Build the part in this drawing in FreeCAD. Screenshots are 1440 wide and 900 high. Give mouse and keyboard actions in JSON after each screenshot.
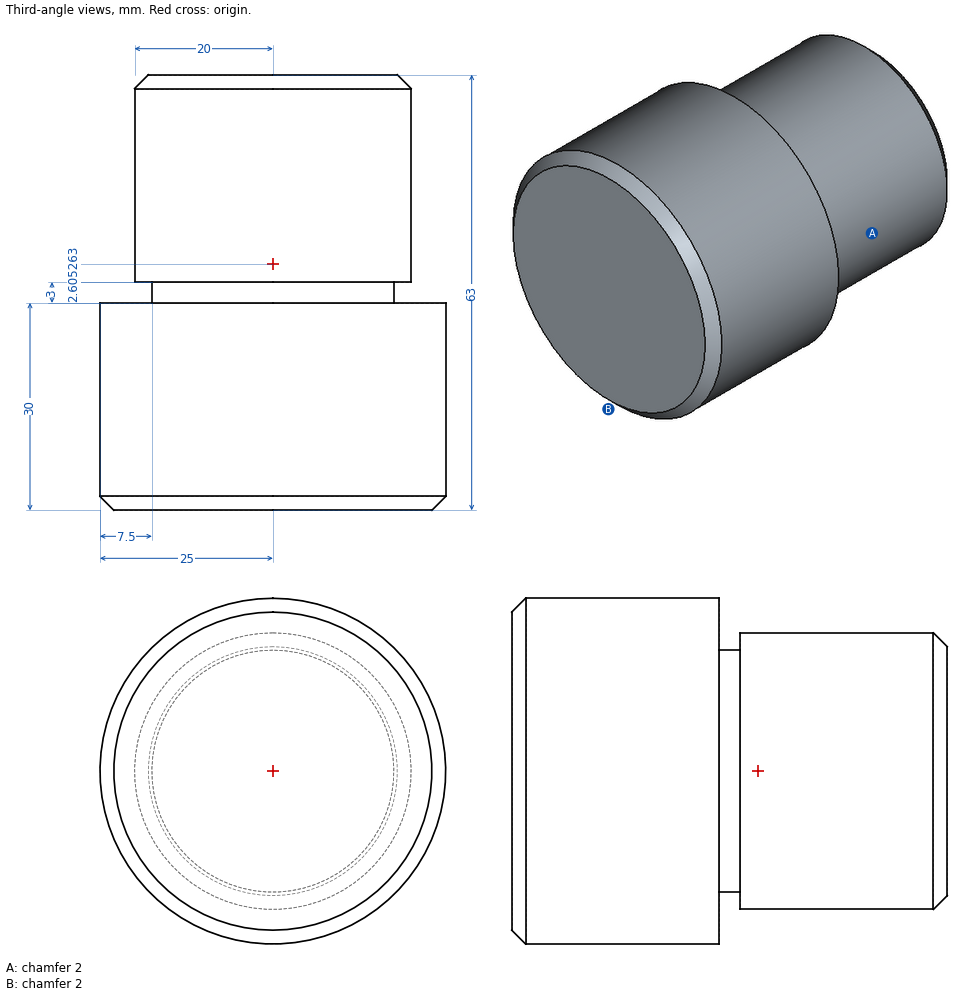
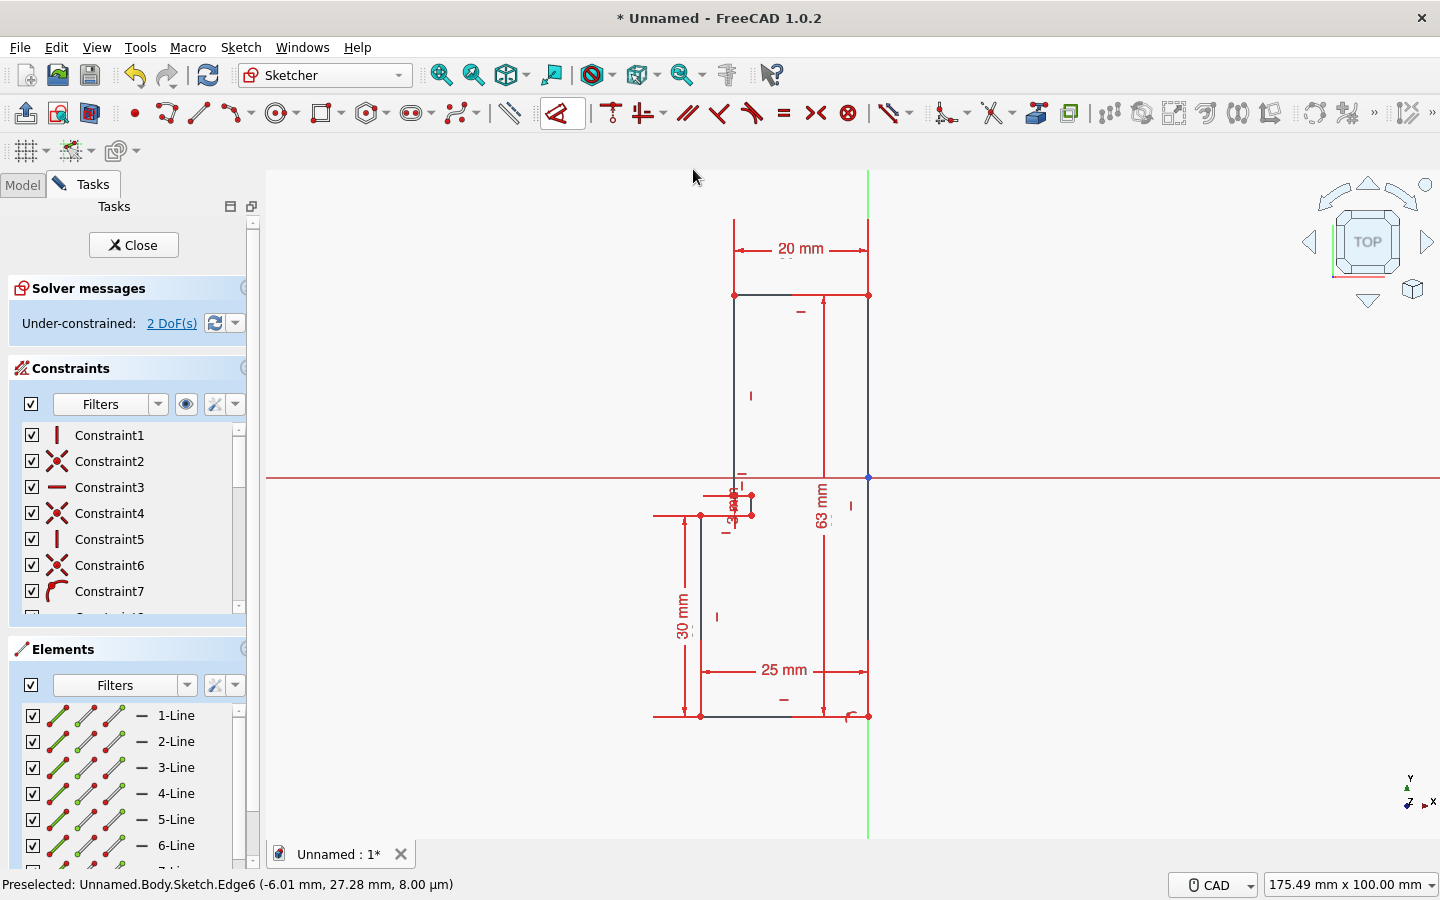
{"action": "left_click", "coordinate": [716, 516]}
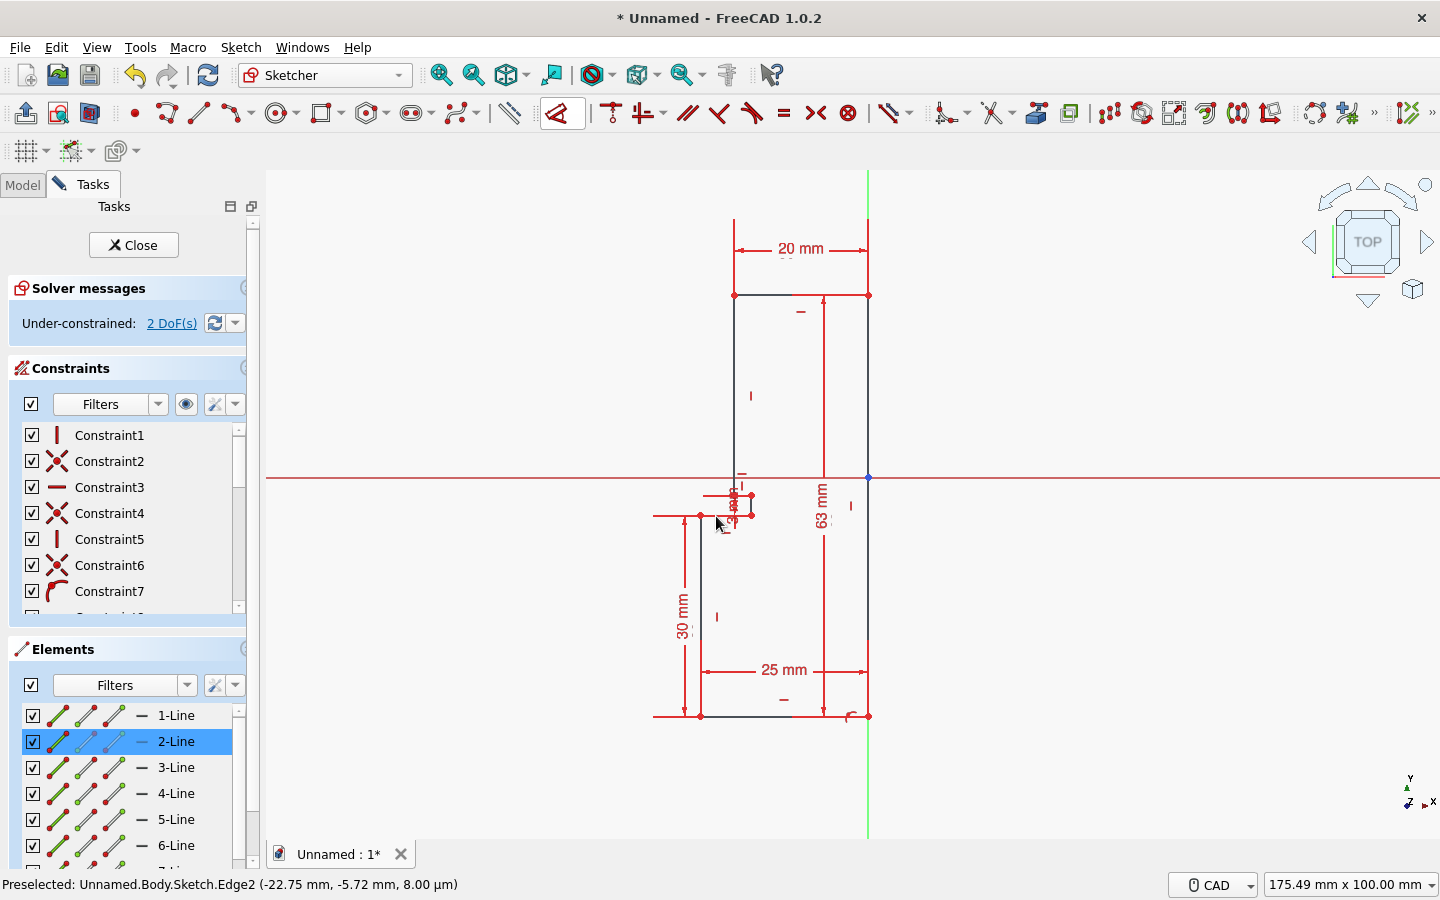
{"action": "key", "text": "l"}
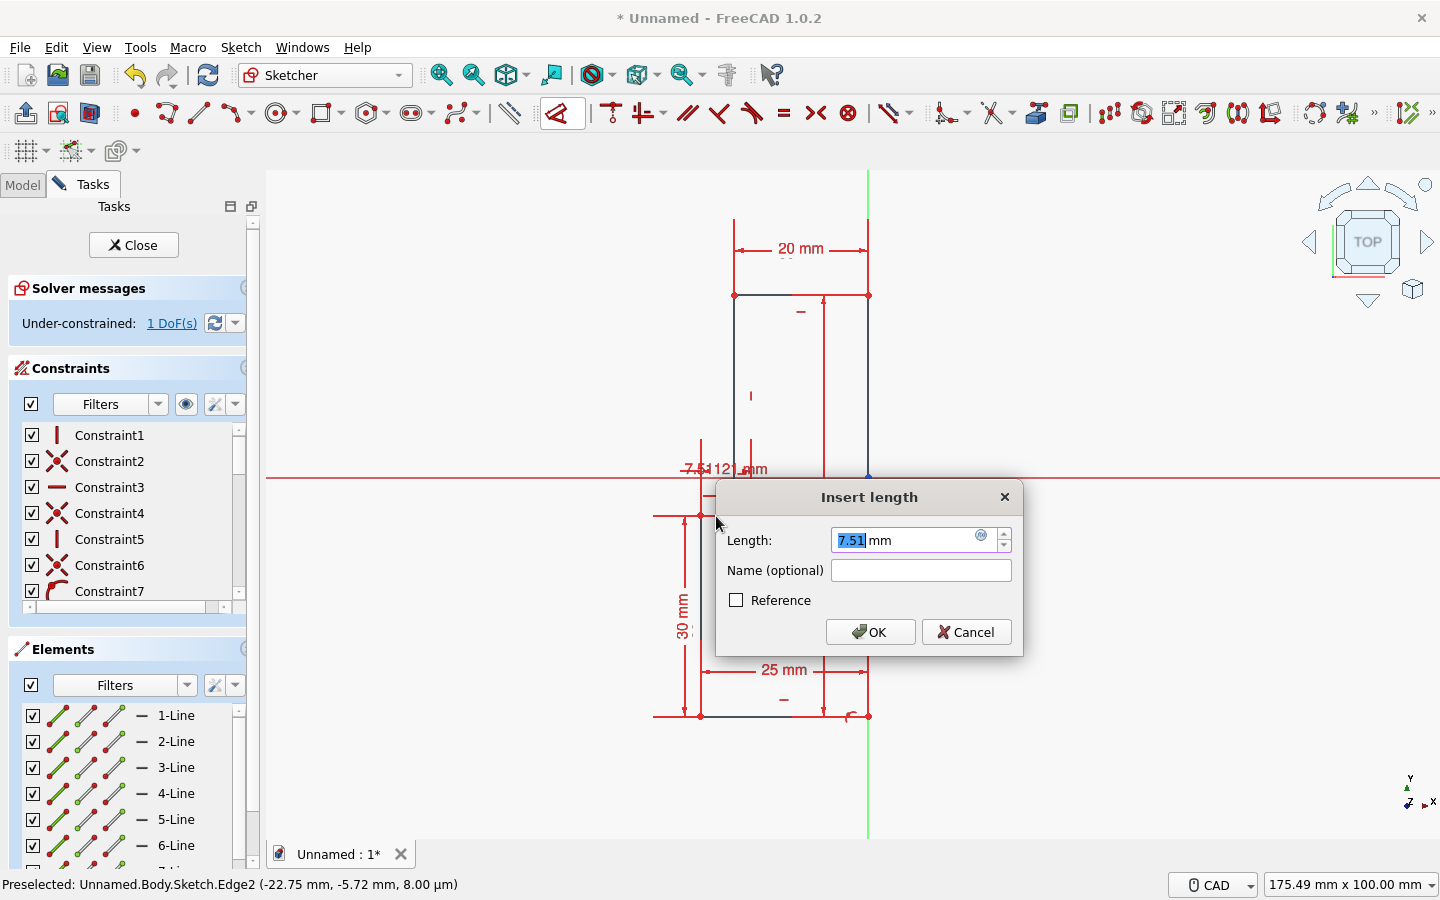
{"action": "type", "text": "7.5"}
{"action": "key", "text": "Return"}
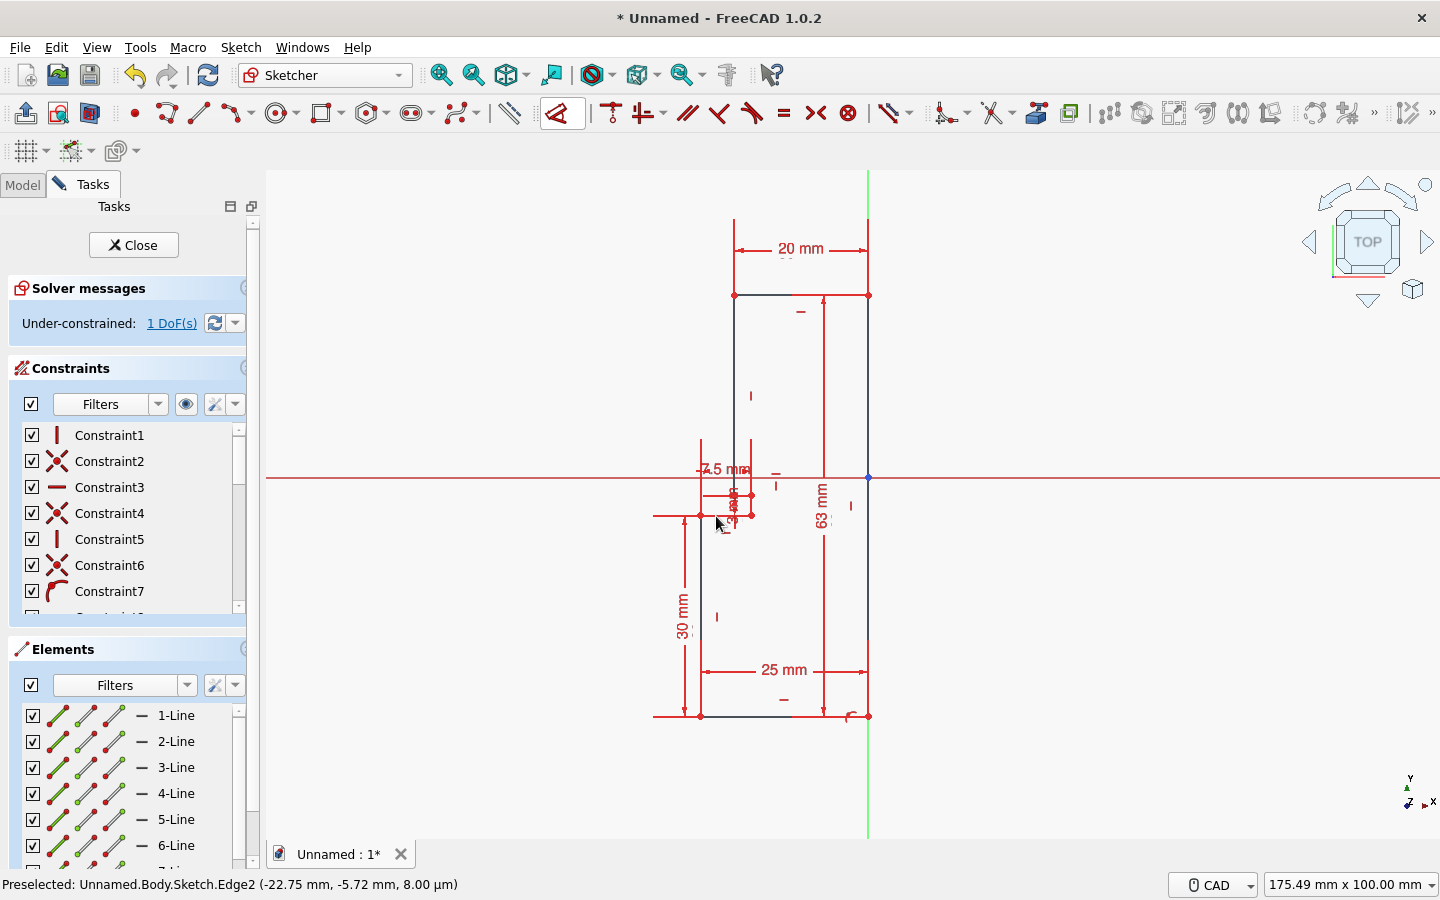
{"action": "scroll", "coordinate": [751, 496], "scroll_direction": "up", "scroll_amount": 5}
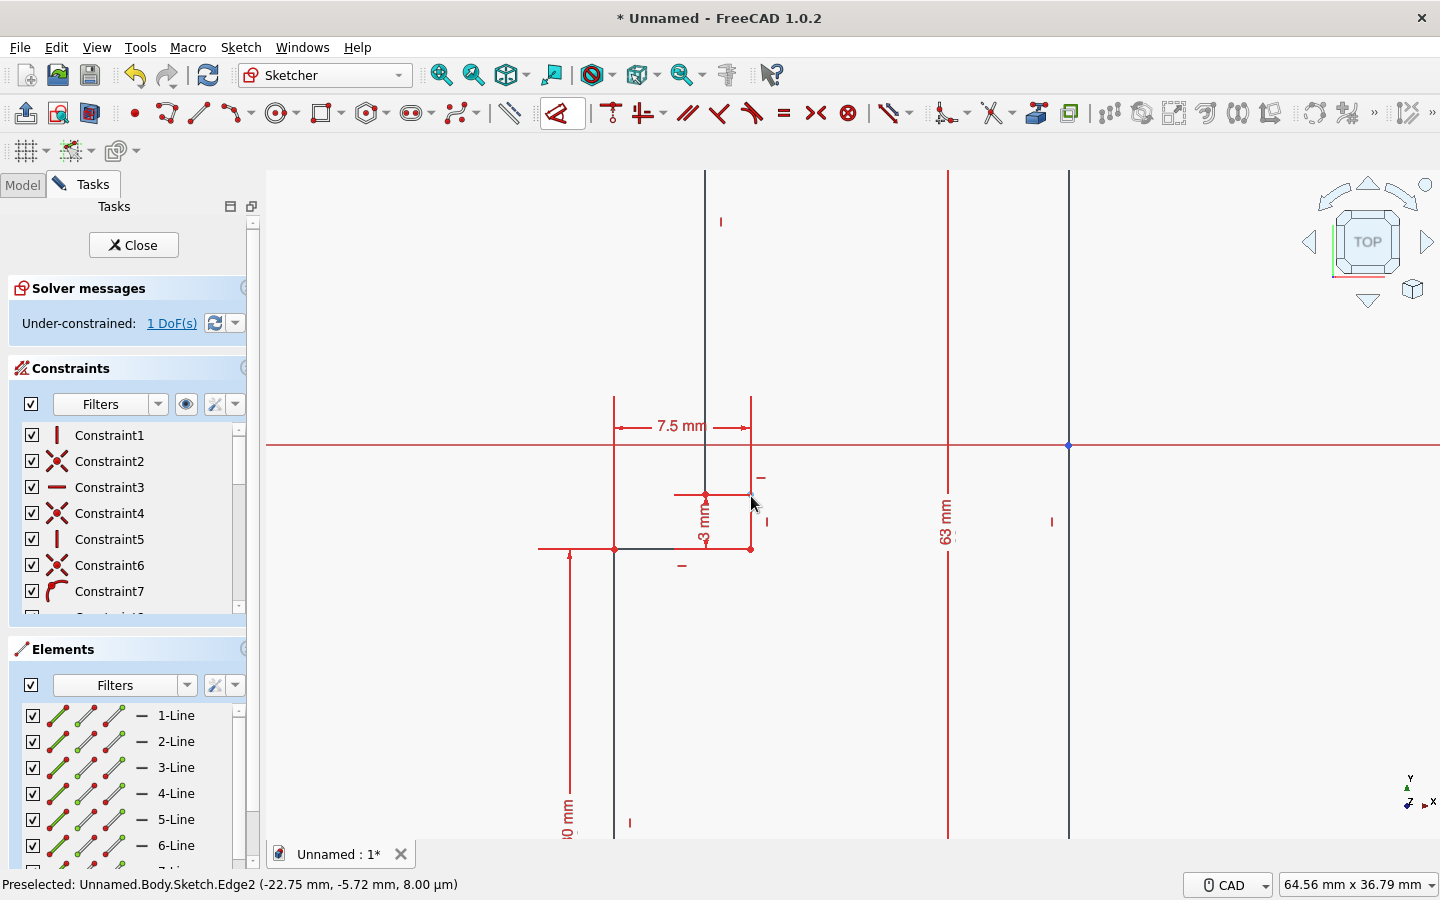
{"action": "left_click", "coordinate": [751, 495]}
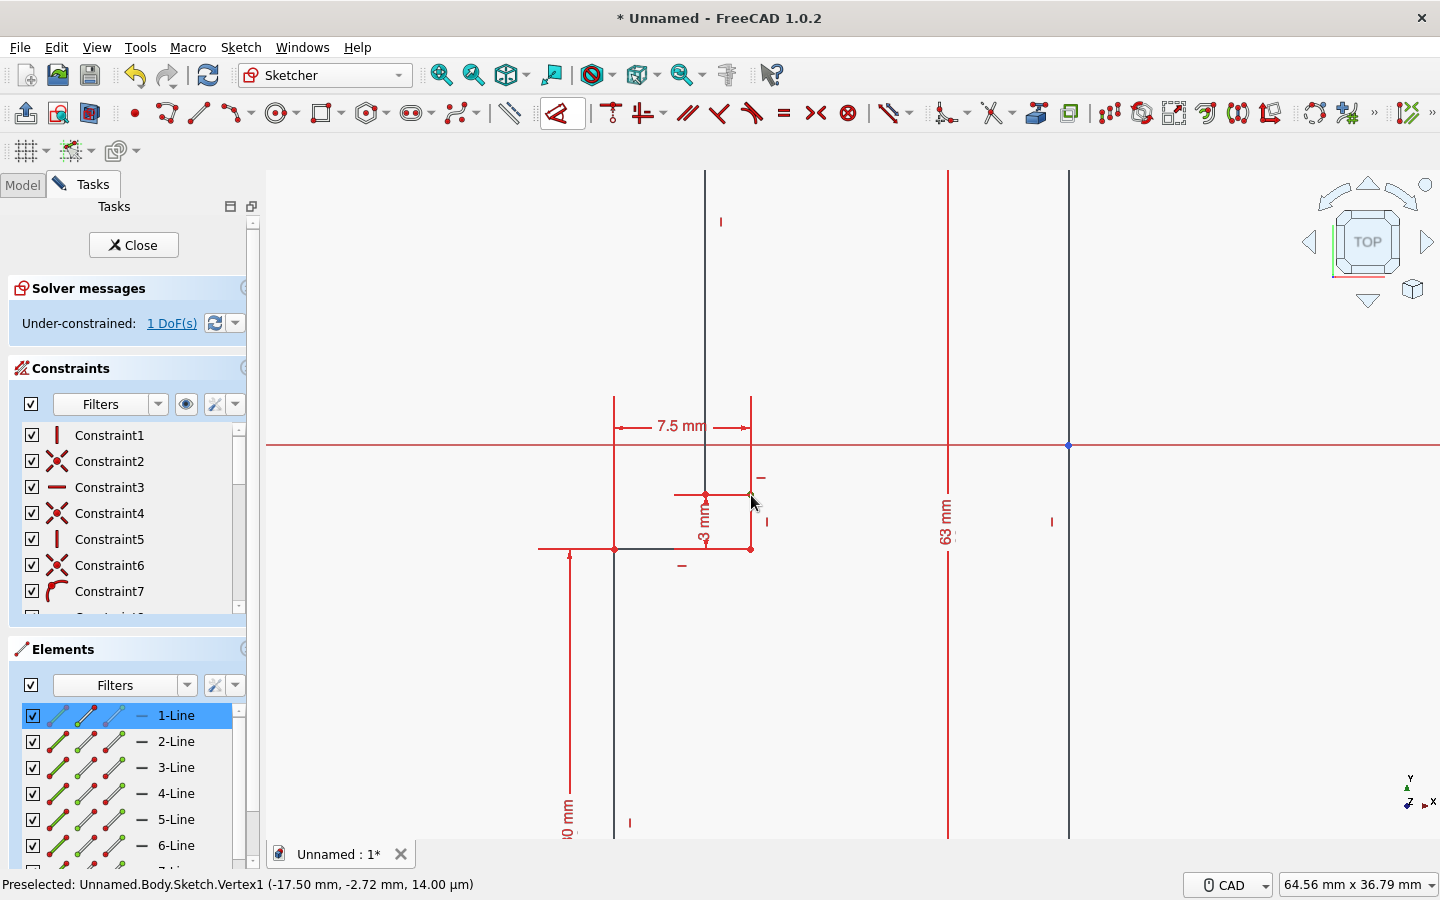
{"action": "key", "text": "i"}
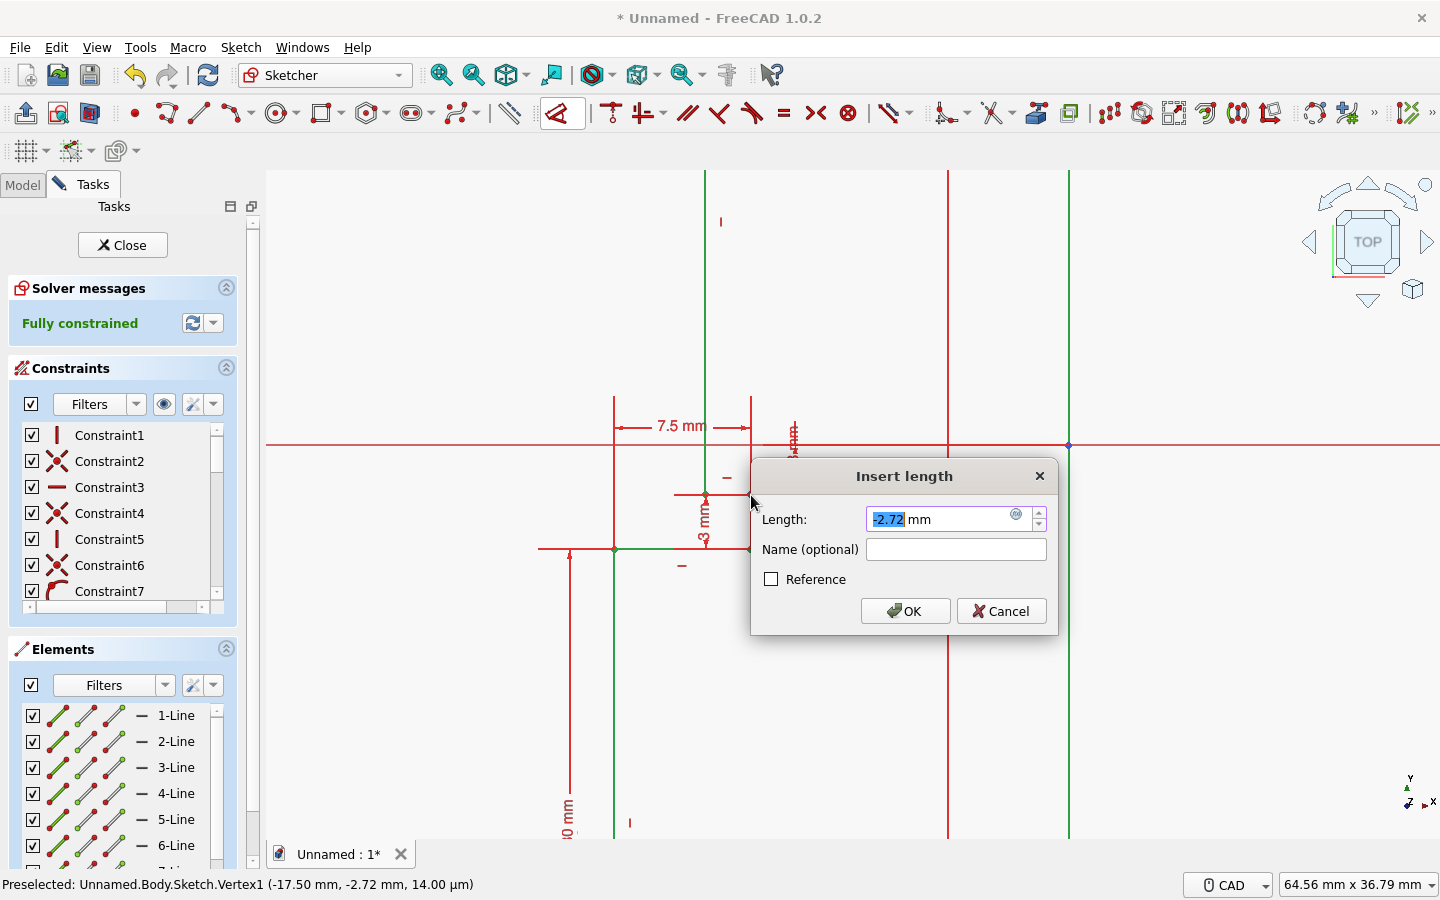
{"action": "type", "text": "-2.605263"}
{"action": "key", "text": "Return"}